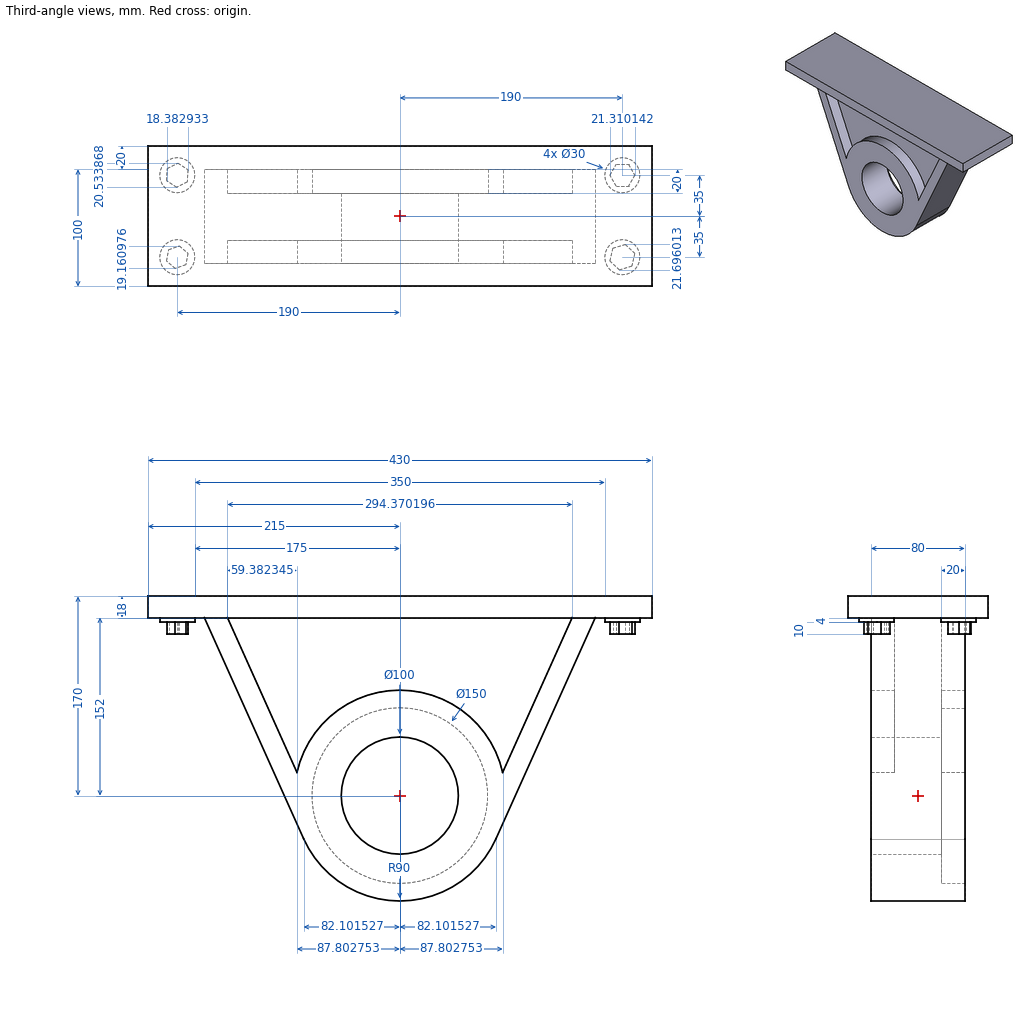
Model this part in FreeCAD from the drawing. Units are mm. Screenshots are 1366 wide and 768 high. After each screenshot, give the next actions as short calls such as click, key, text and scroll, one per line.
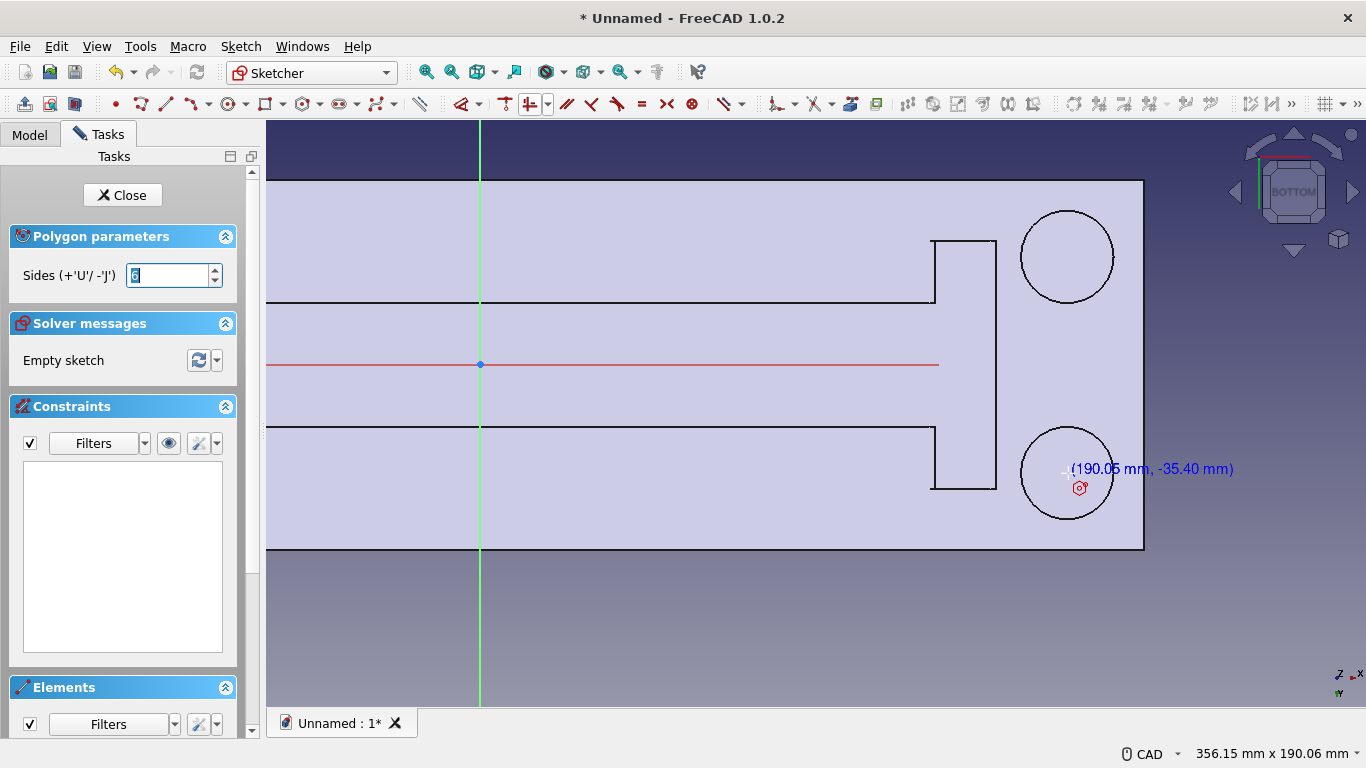
click(1067, 473)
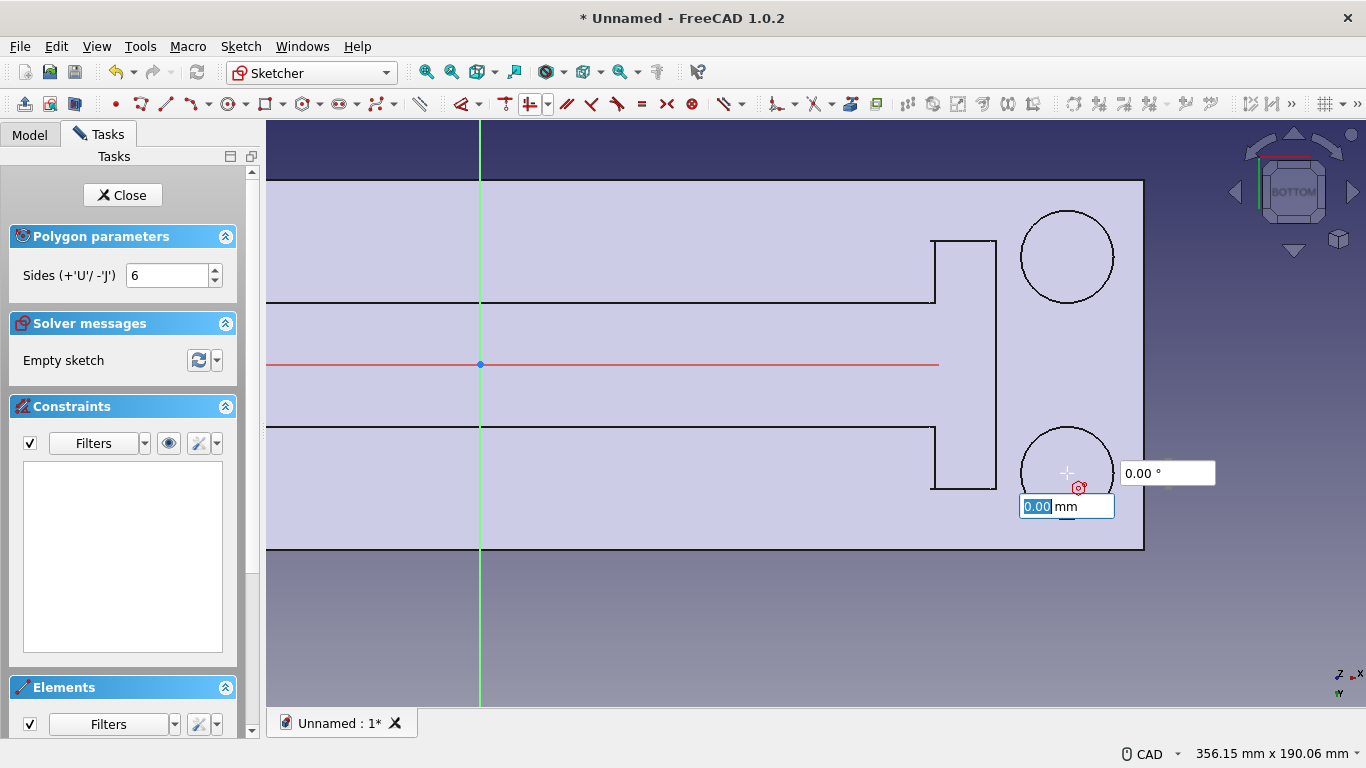
click(1034, 473)
right_click(1034, 473)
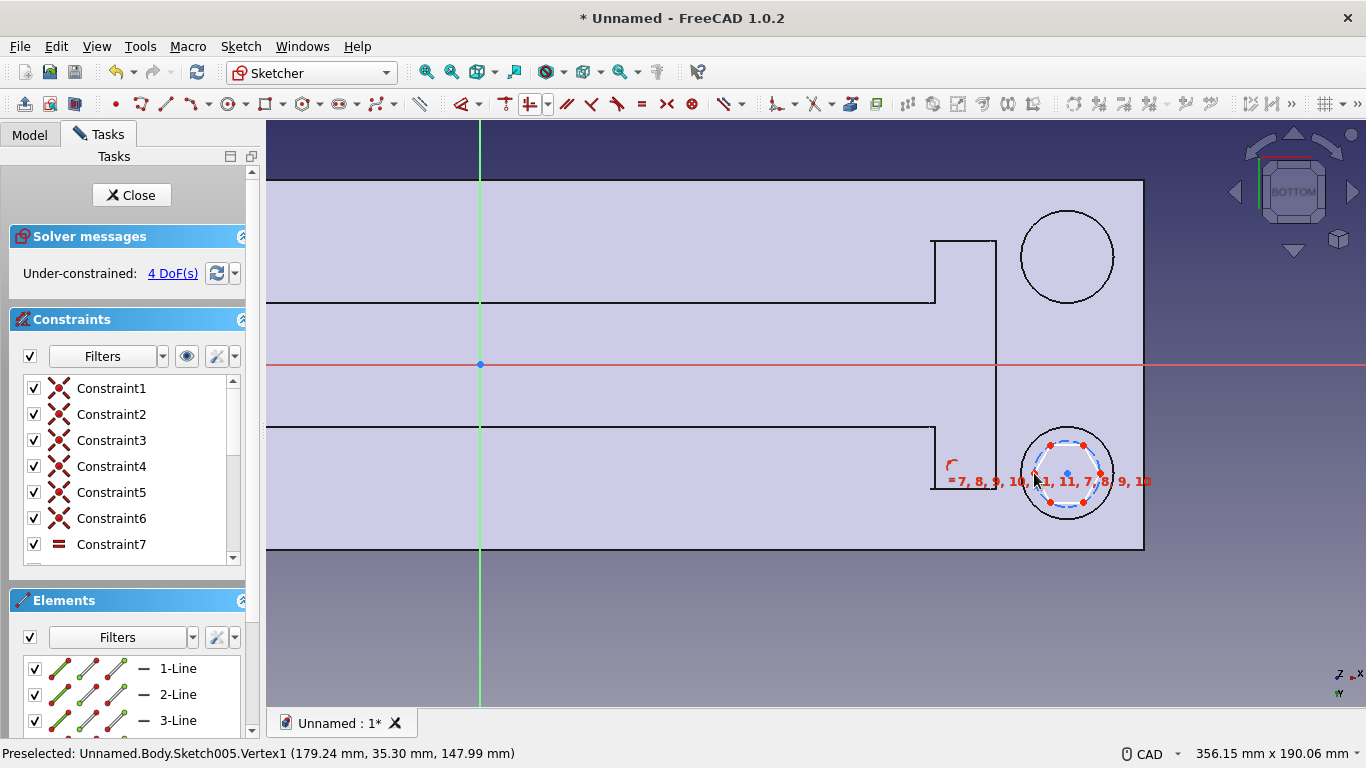
click(302, 104)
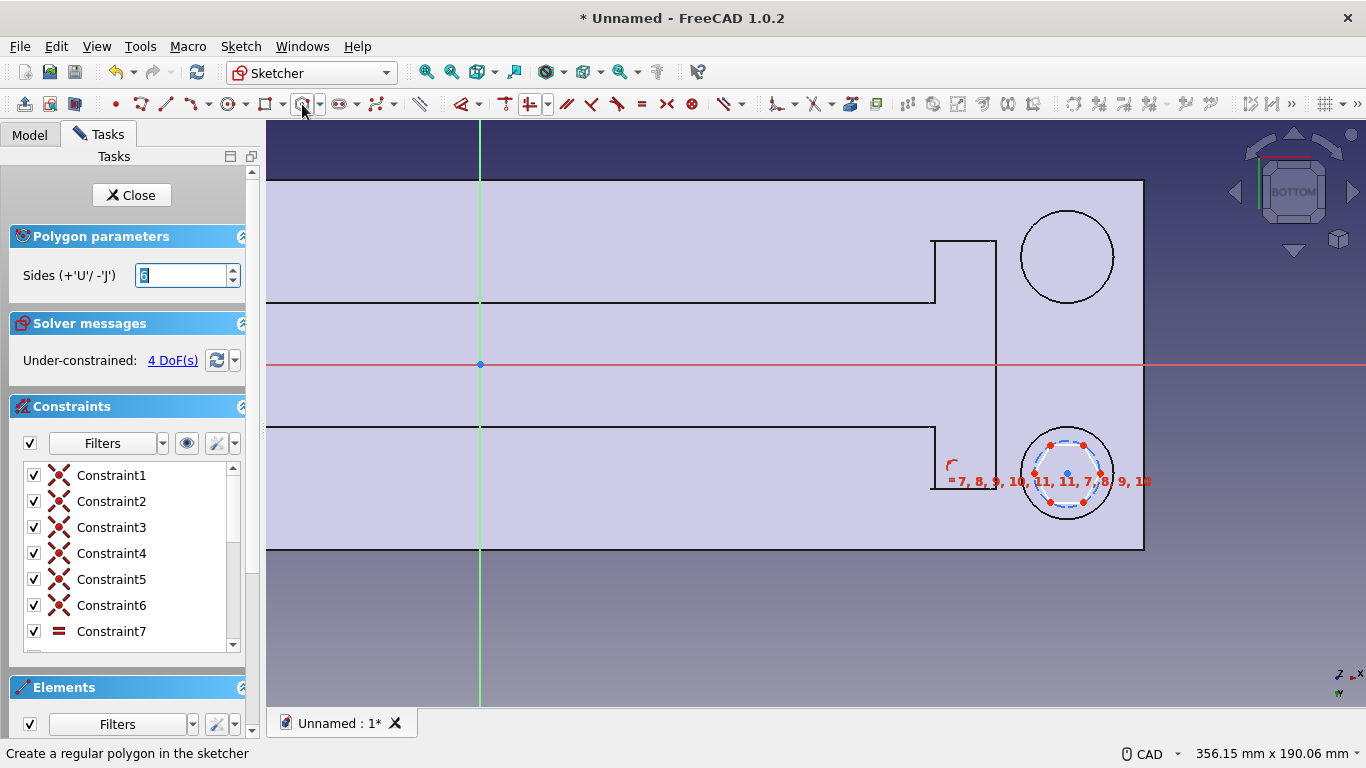
click(1067, 257)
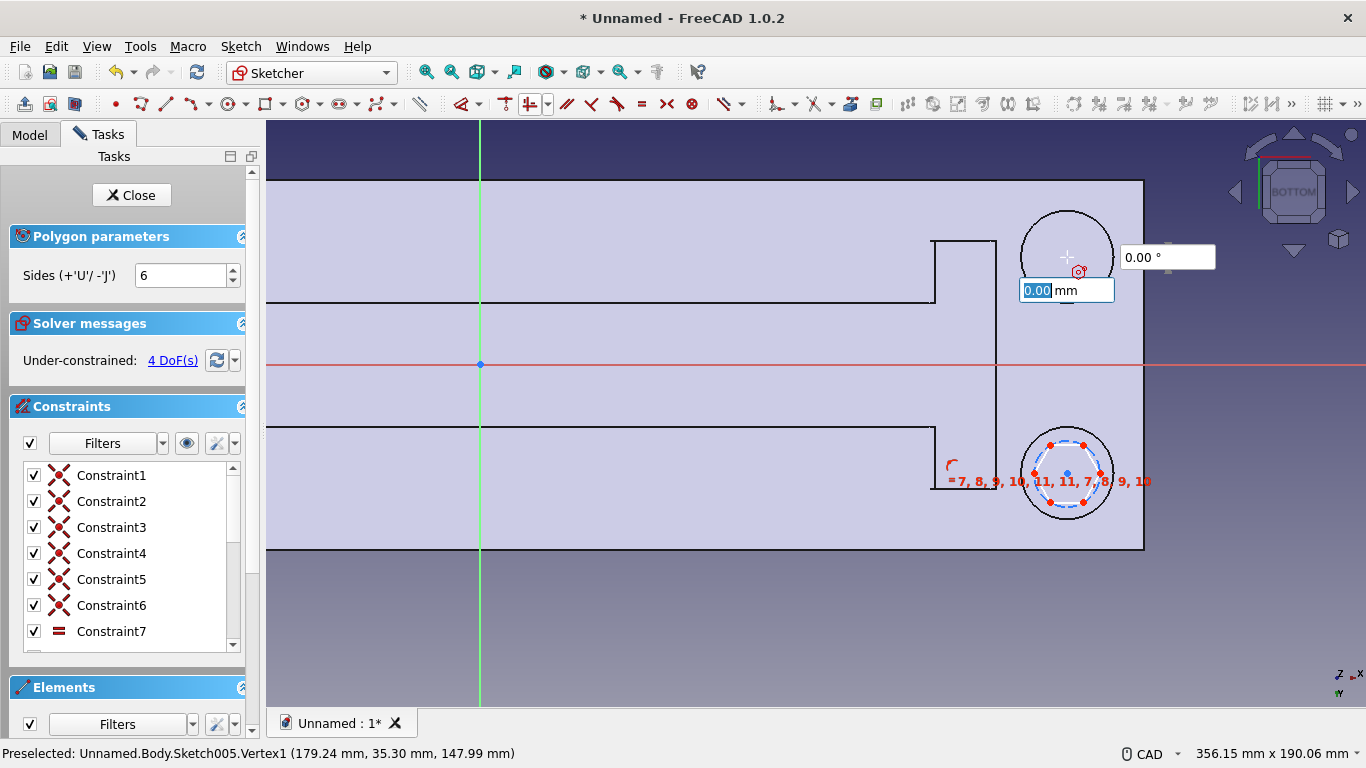
click(1059, 223)
right_click(1059, 223)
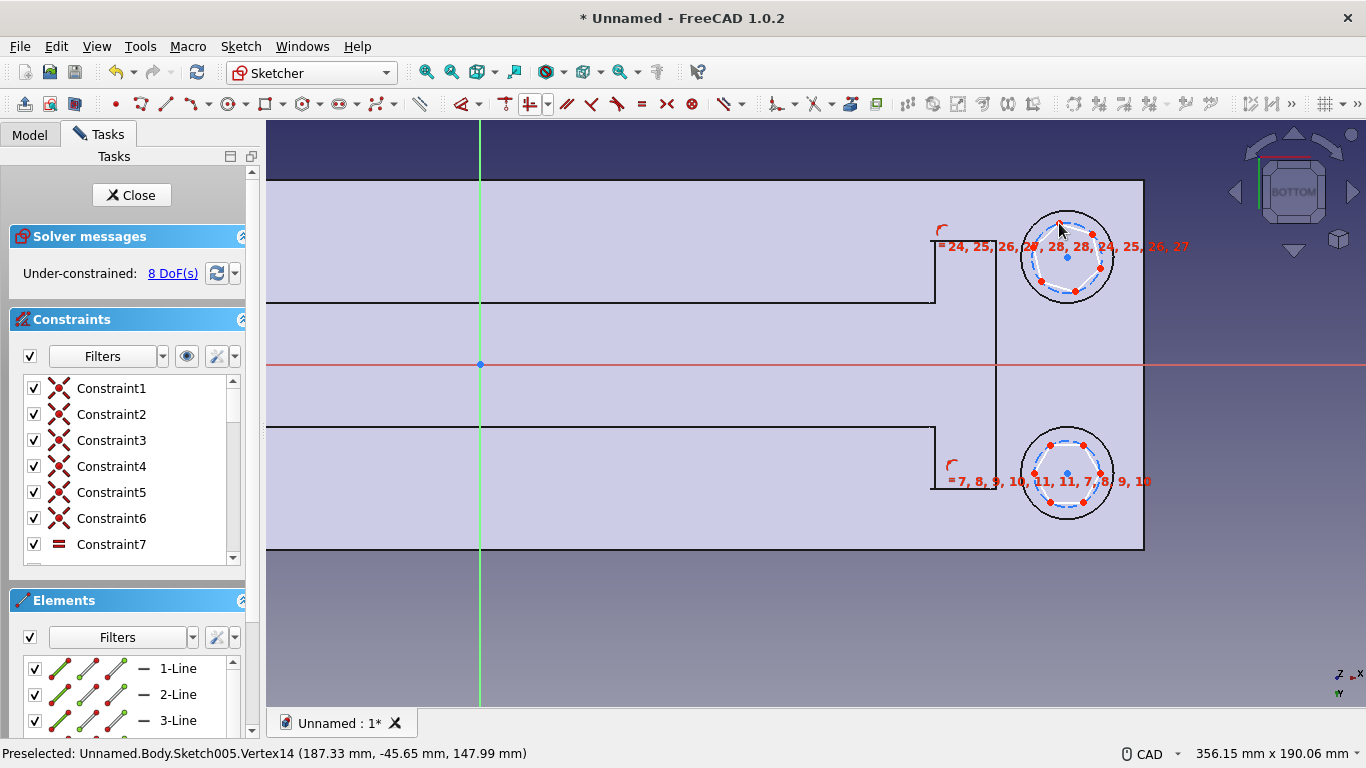
click(302, 104)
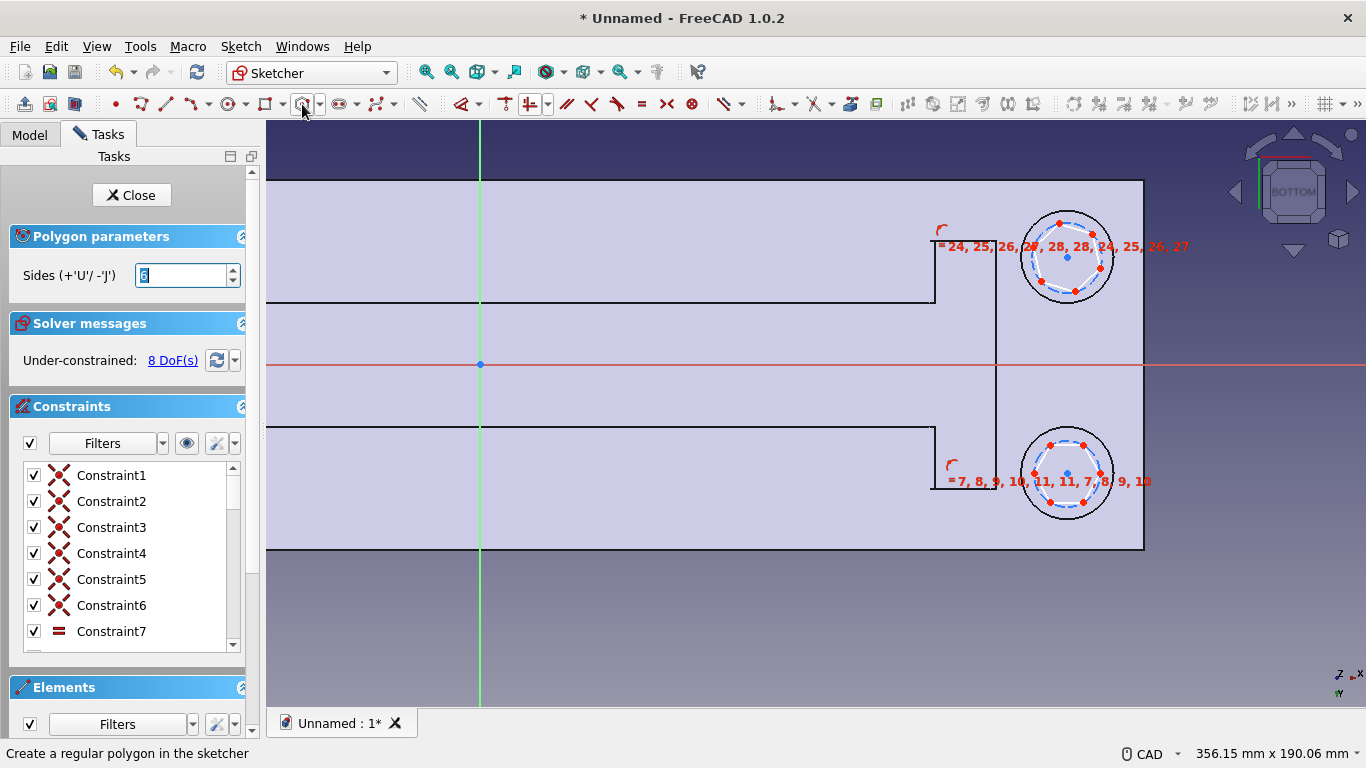
scroll(1070, 474, down, 3)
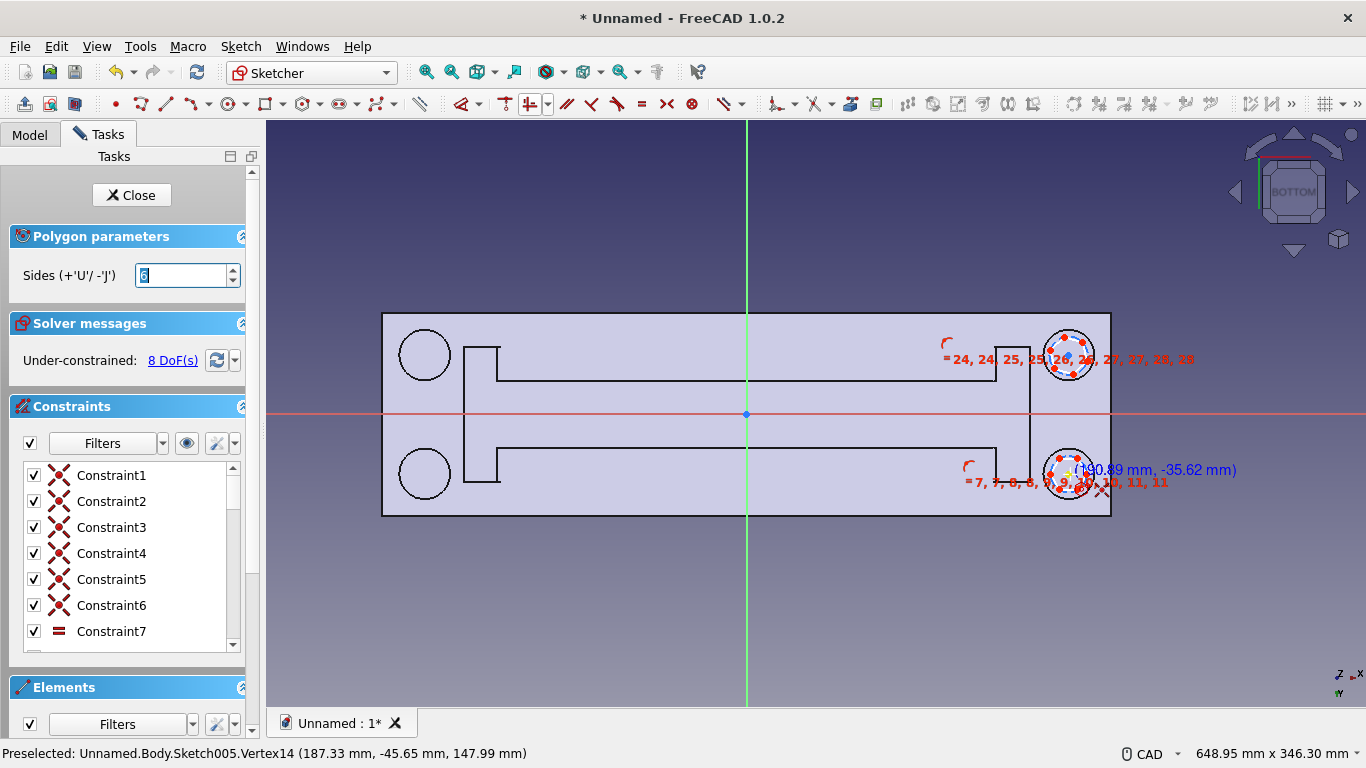
scroll(425, 474, up, 3)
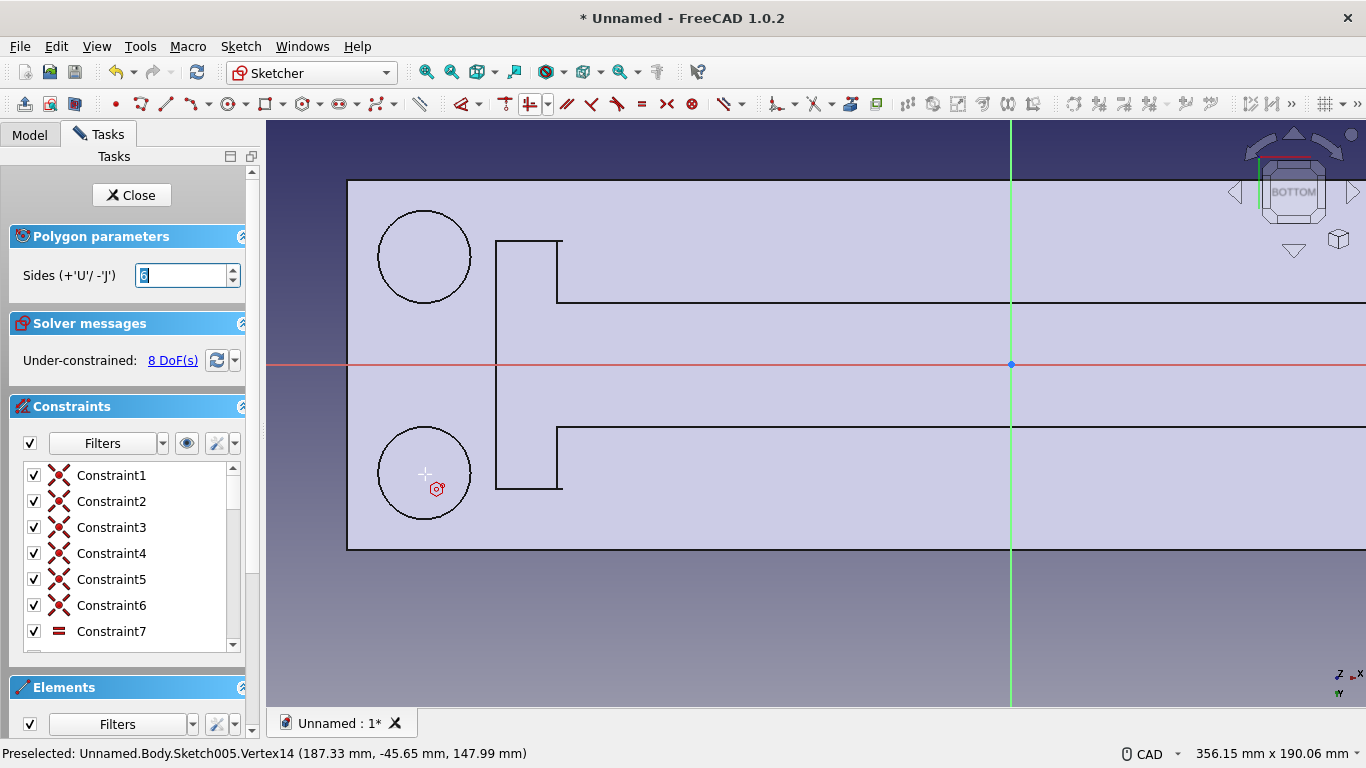
click(424, 473)